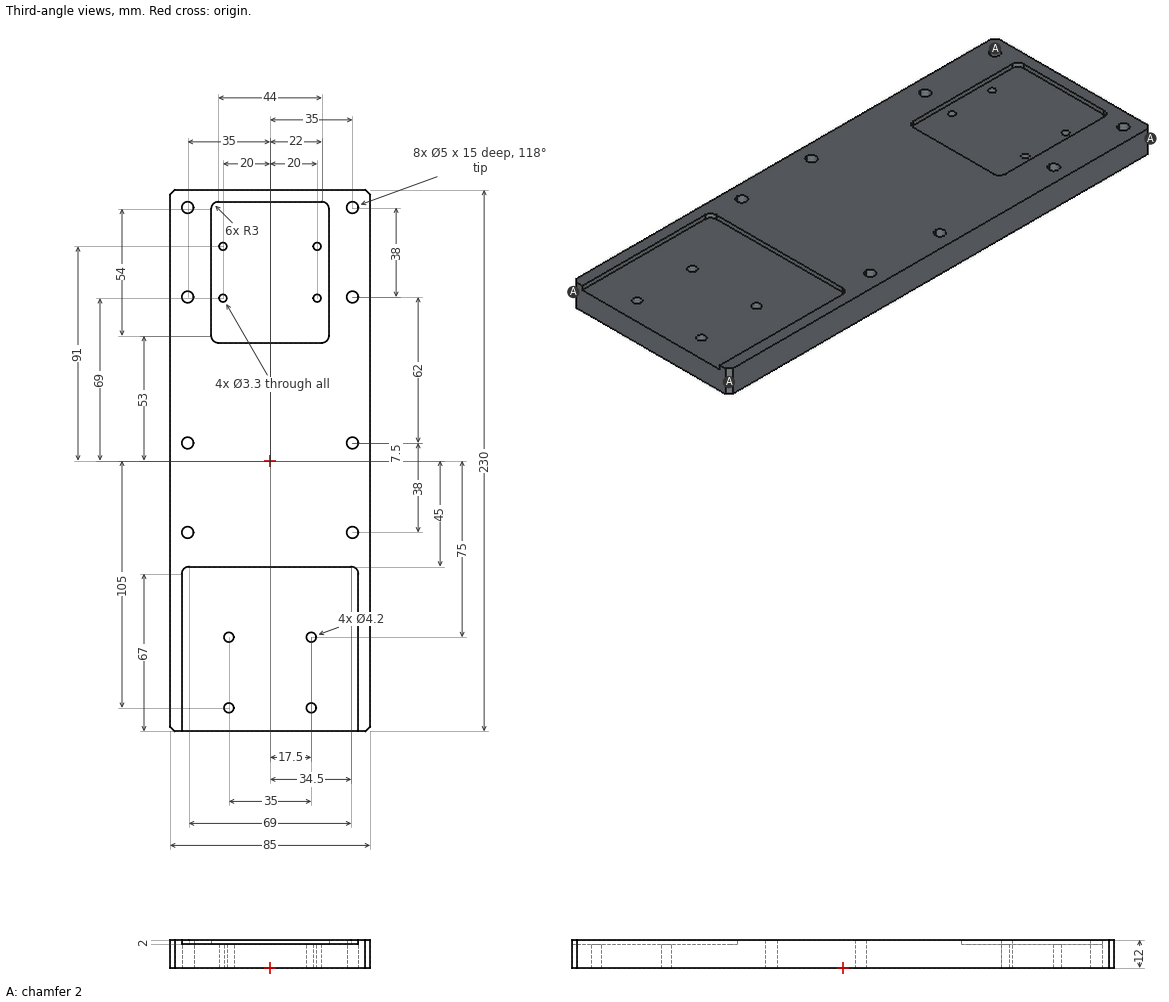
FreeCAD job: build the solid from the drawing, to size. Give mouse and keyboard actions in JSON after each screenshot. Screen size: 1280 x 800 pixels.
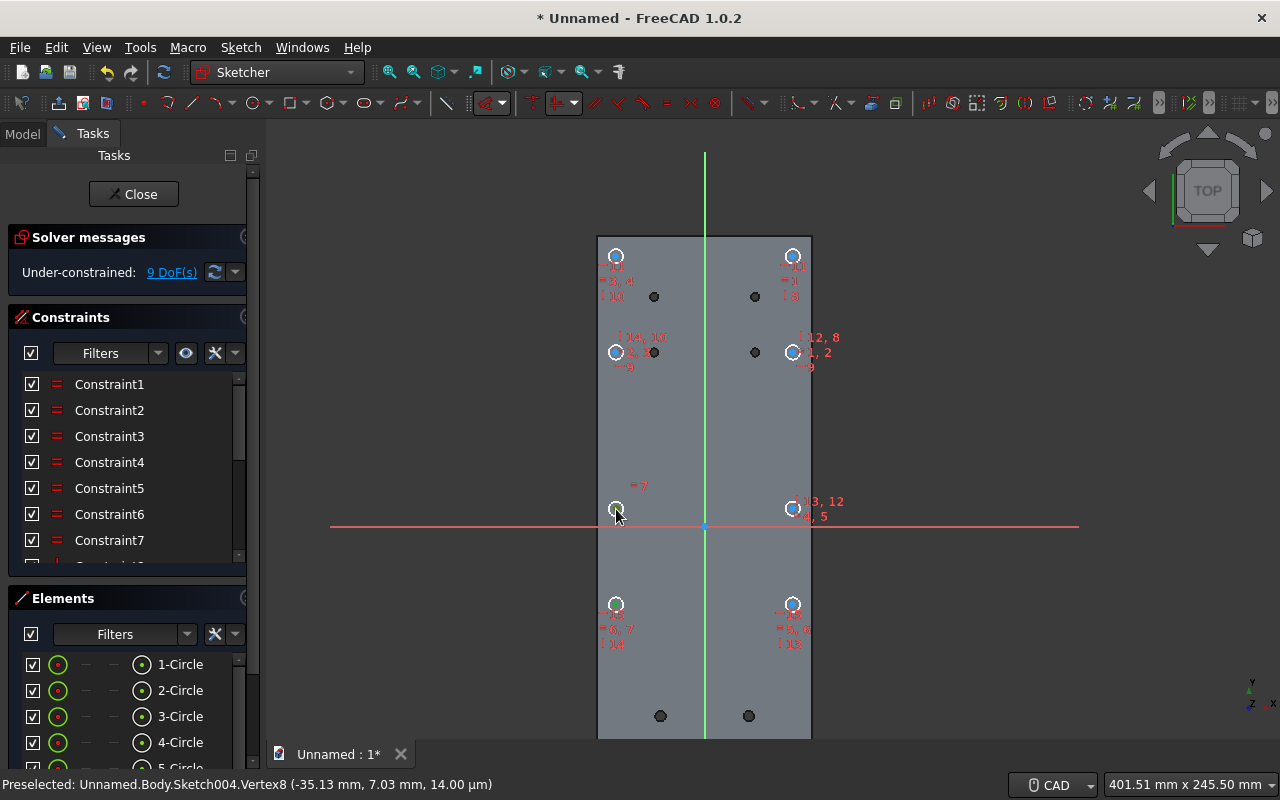
{"action": "key", "text": "v"}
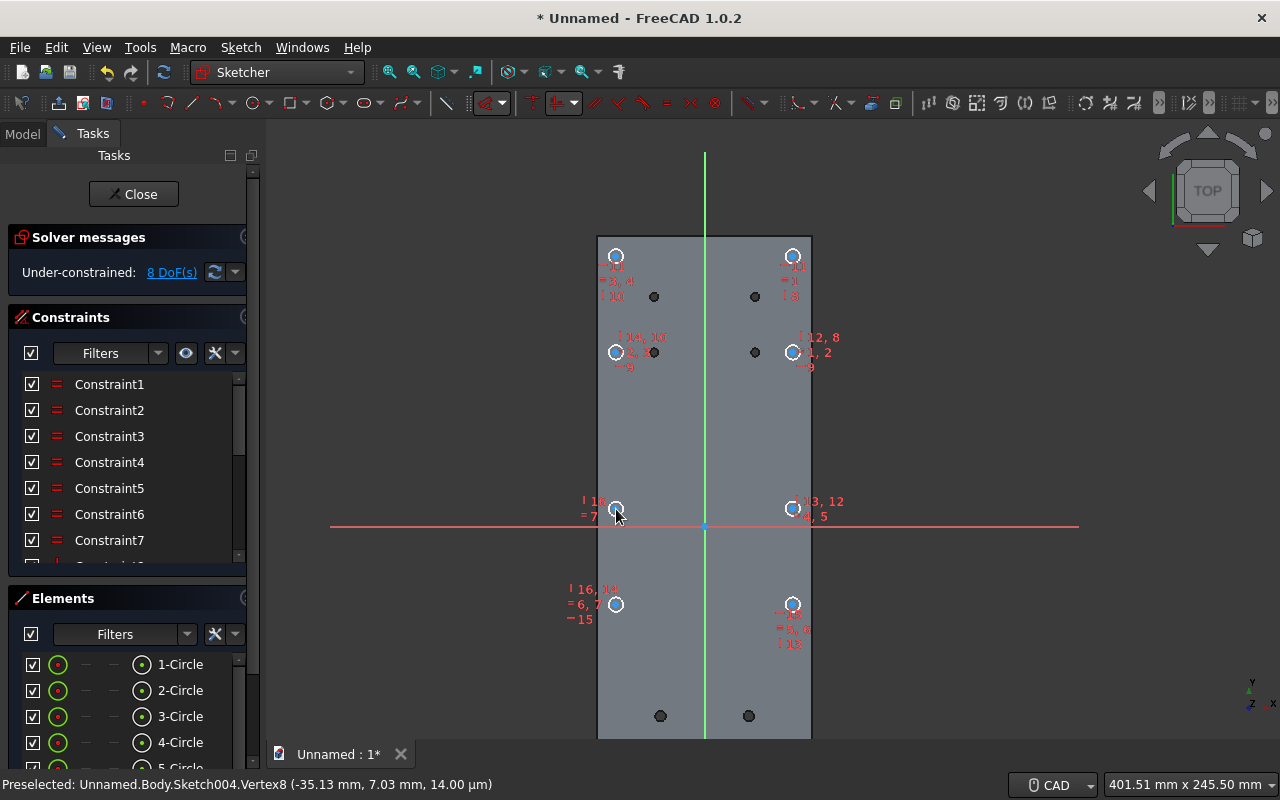
{"action": "left_click", "coordinate": [793, 509]}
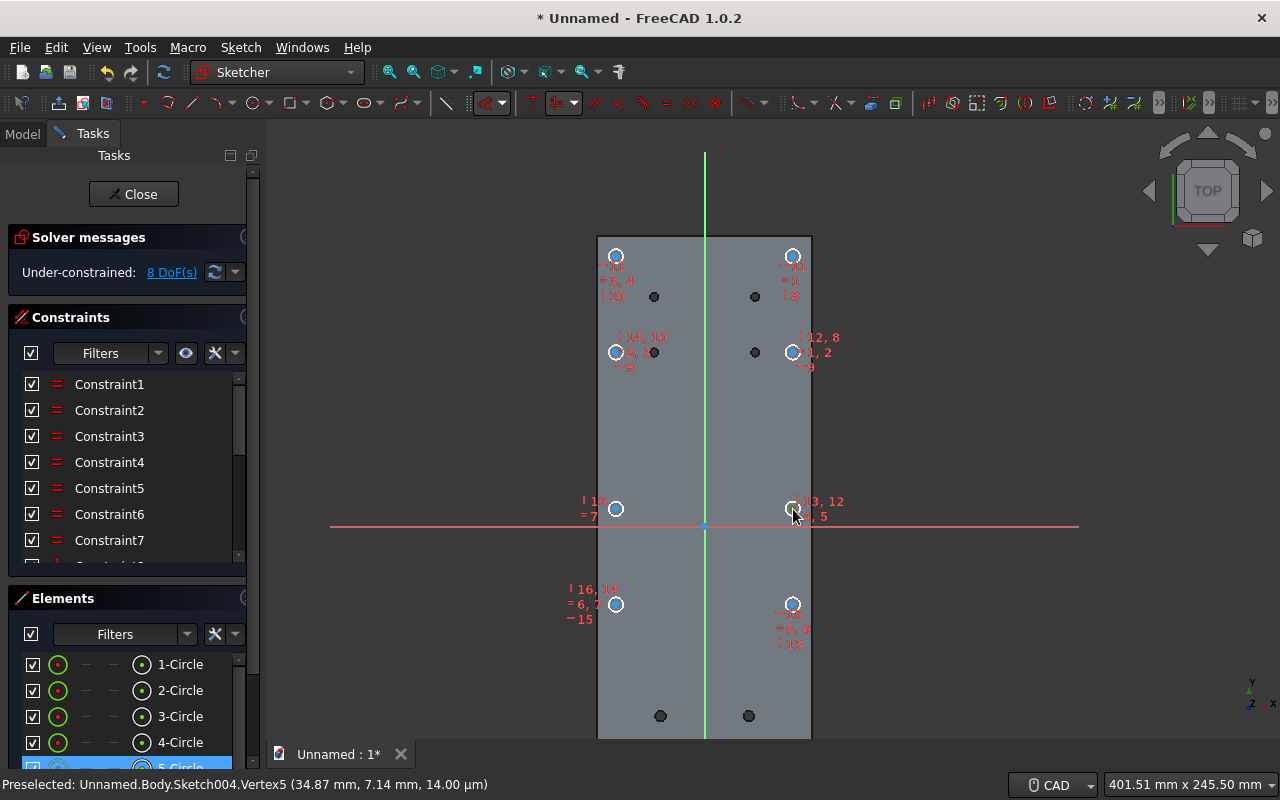
{"action": "left_click", "coordinate": [616, 509]}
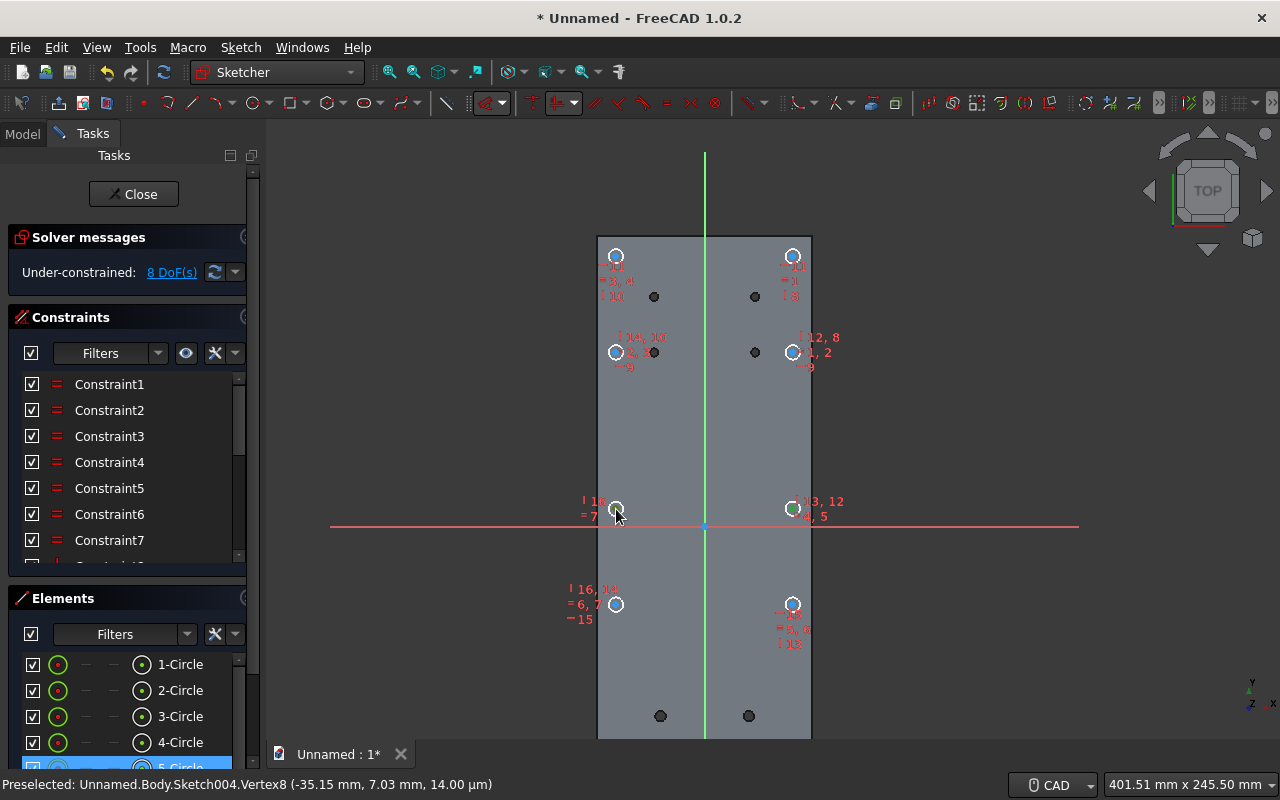
{"action": "key", "text": "h"}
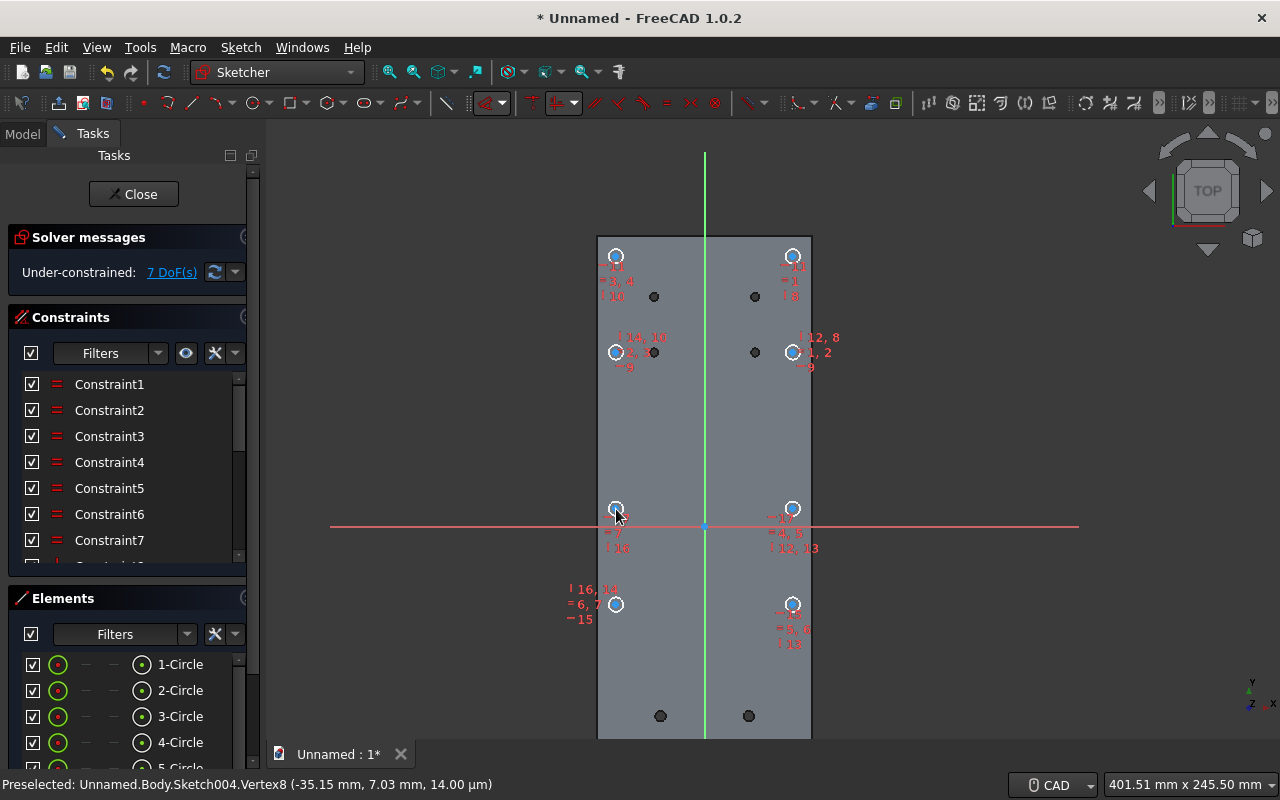
{"action": "scroll", "coordinate": [798, 251], "scroll_direction": "up", "scroll_amount": 6}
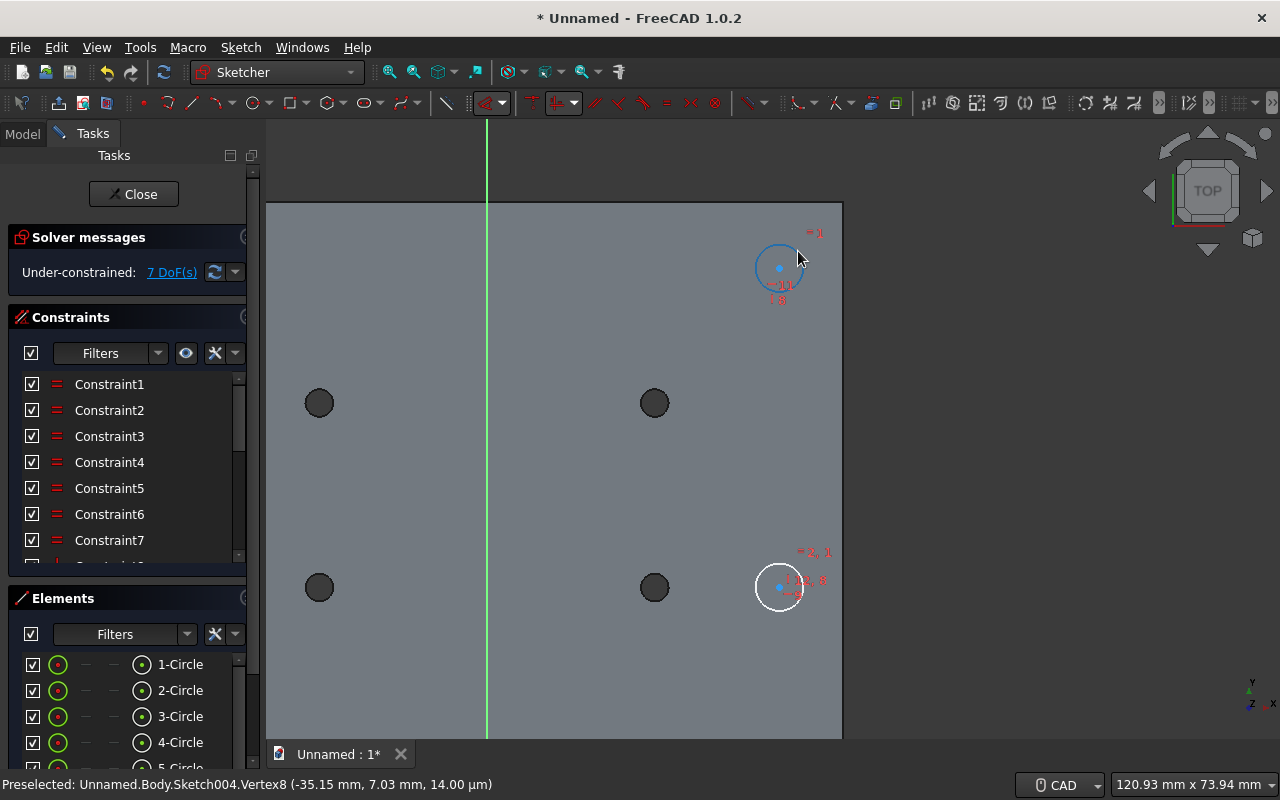
{"action": "left_click", "coordinate": [796, 251]}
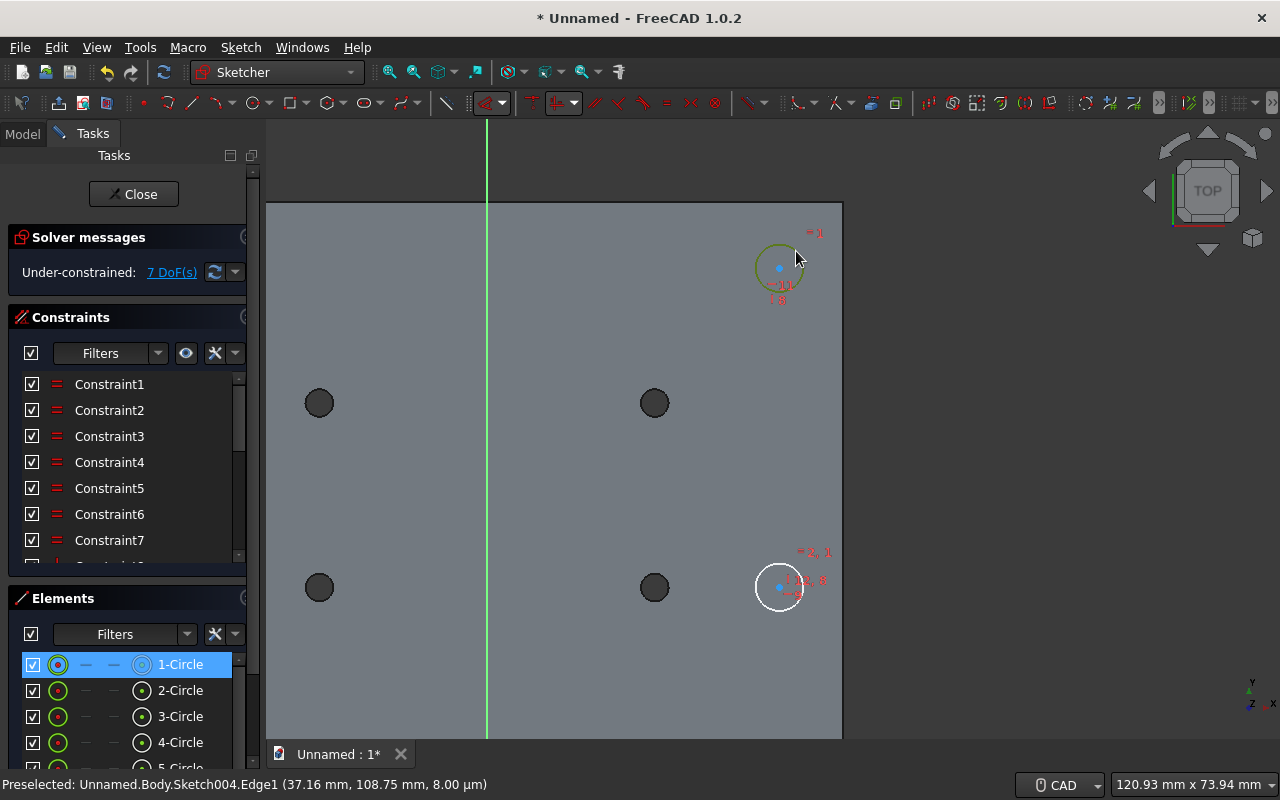
{"action": "key", "text": "k o"}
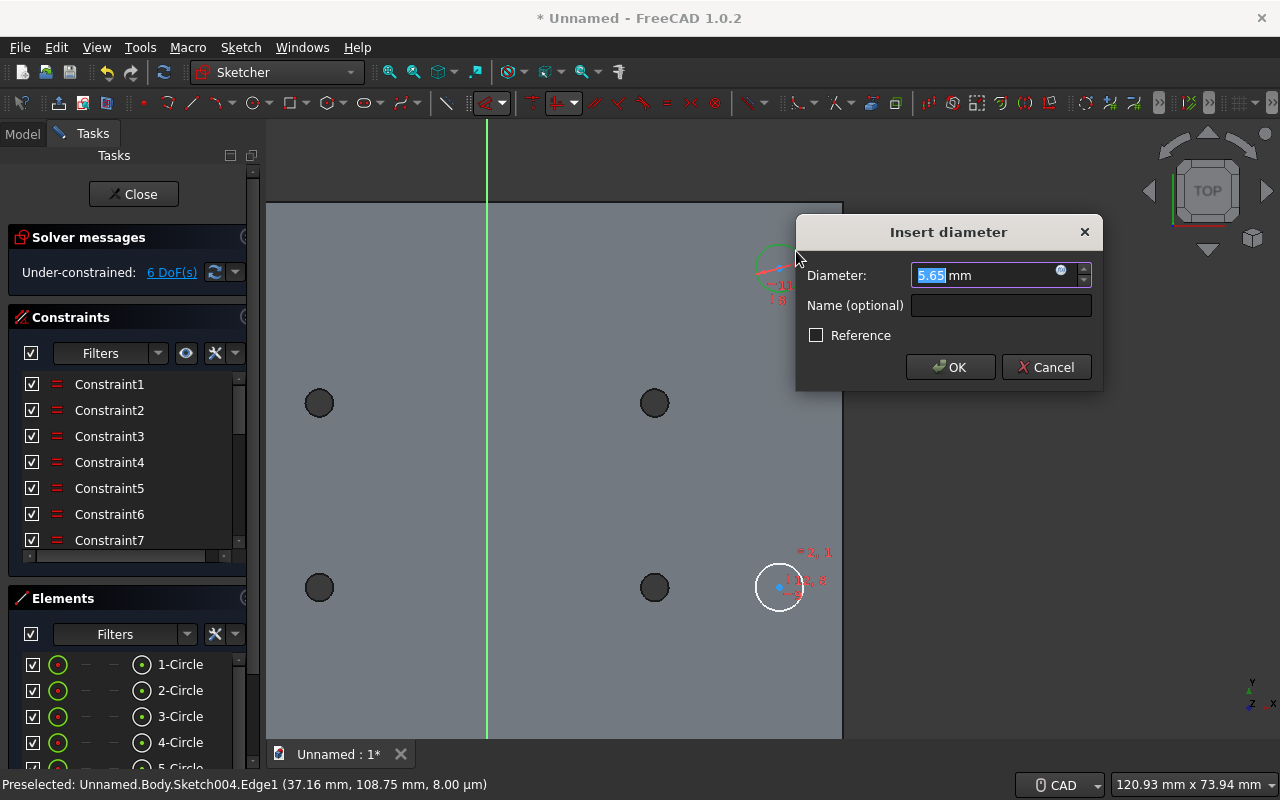
{"action": "type", "text": "5"}
{"action": "key", "text": "Return"}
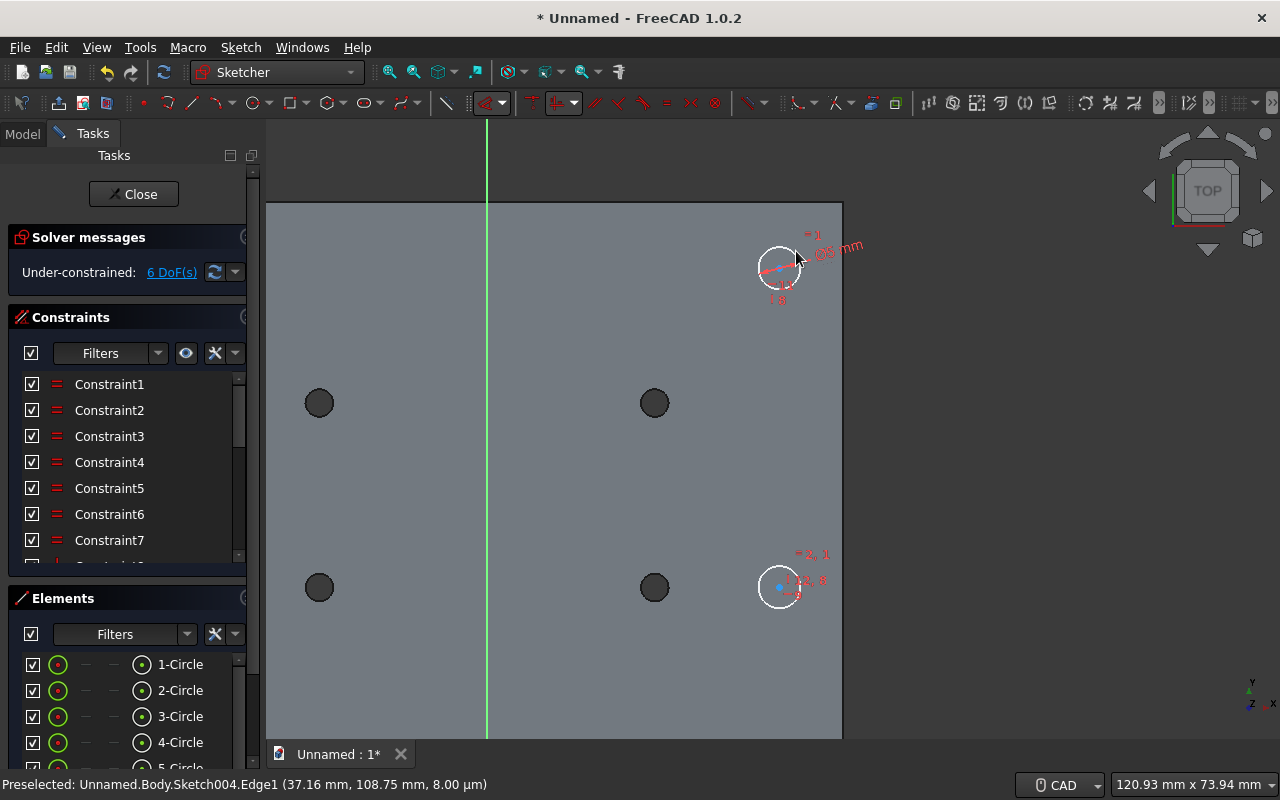
{"action": "scroll", "coordinate": [798, 250], "scroll_direction": "down", "scroll_amount": 6}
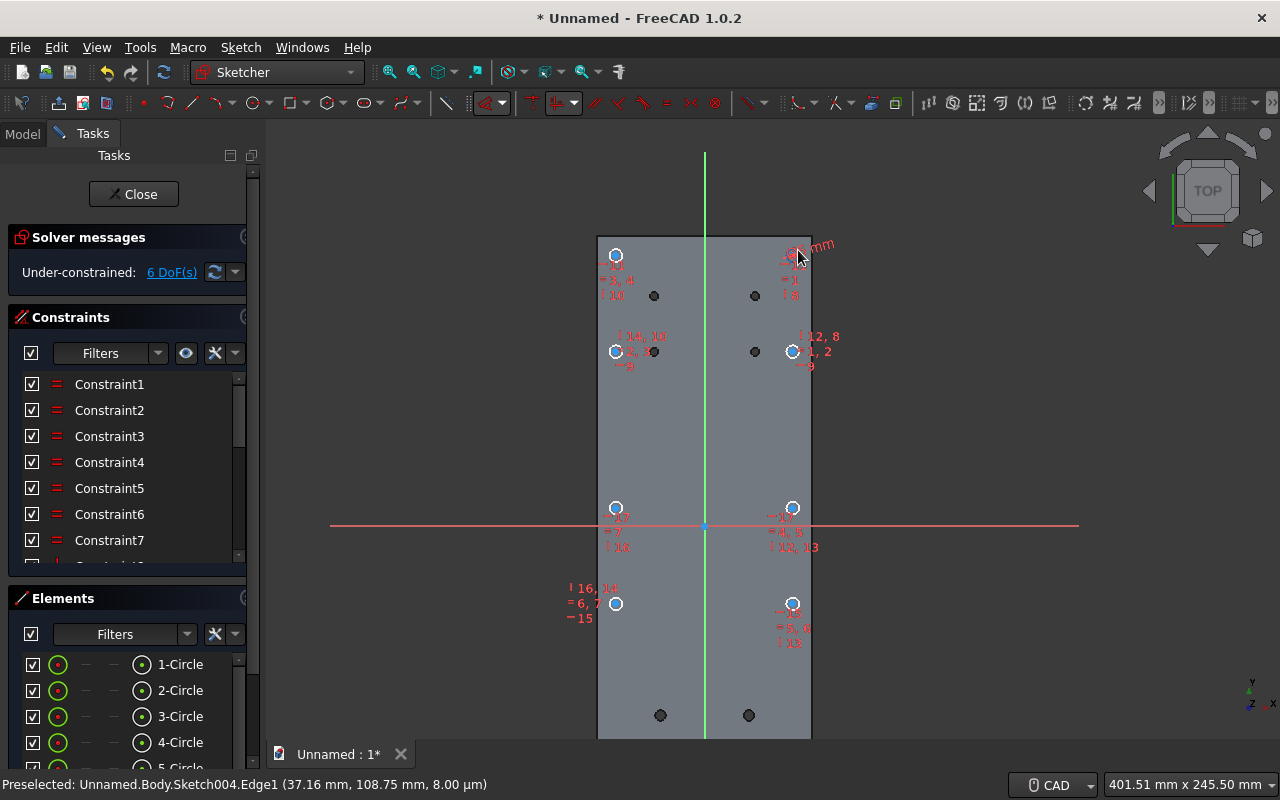
{"action": "left_click", "coordinate": [793, 256]}